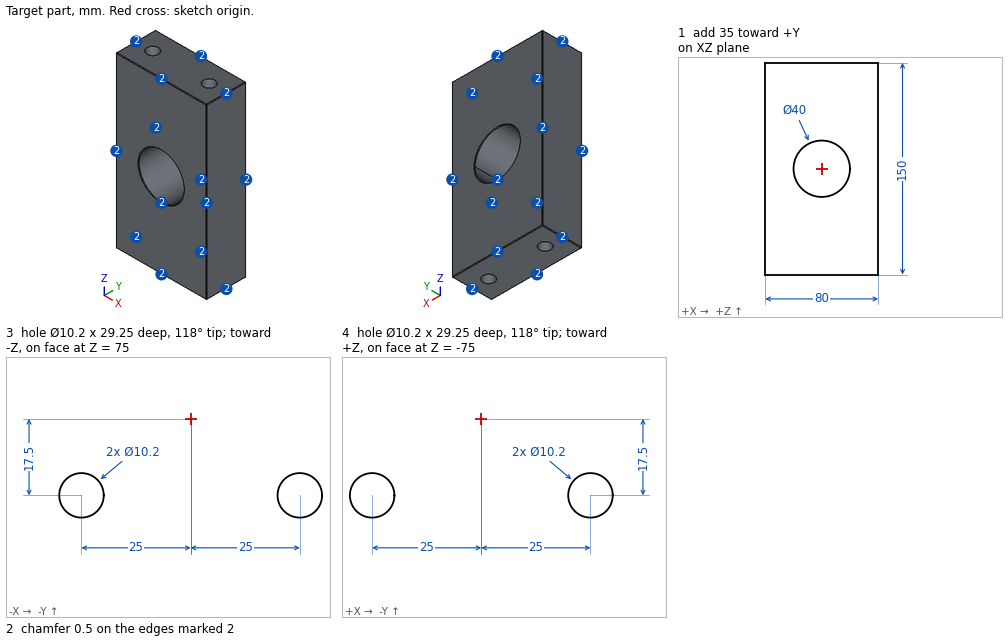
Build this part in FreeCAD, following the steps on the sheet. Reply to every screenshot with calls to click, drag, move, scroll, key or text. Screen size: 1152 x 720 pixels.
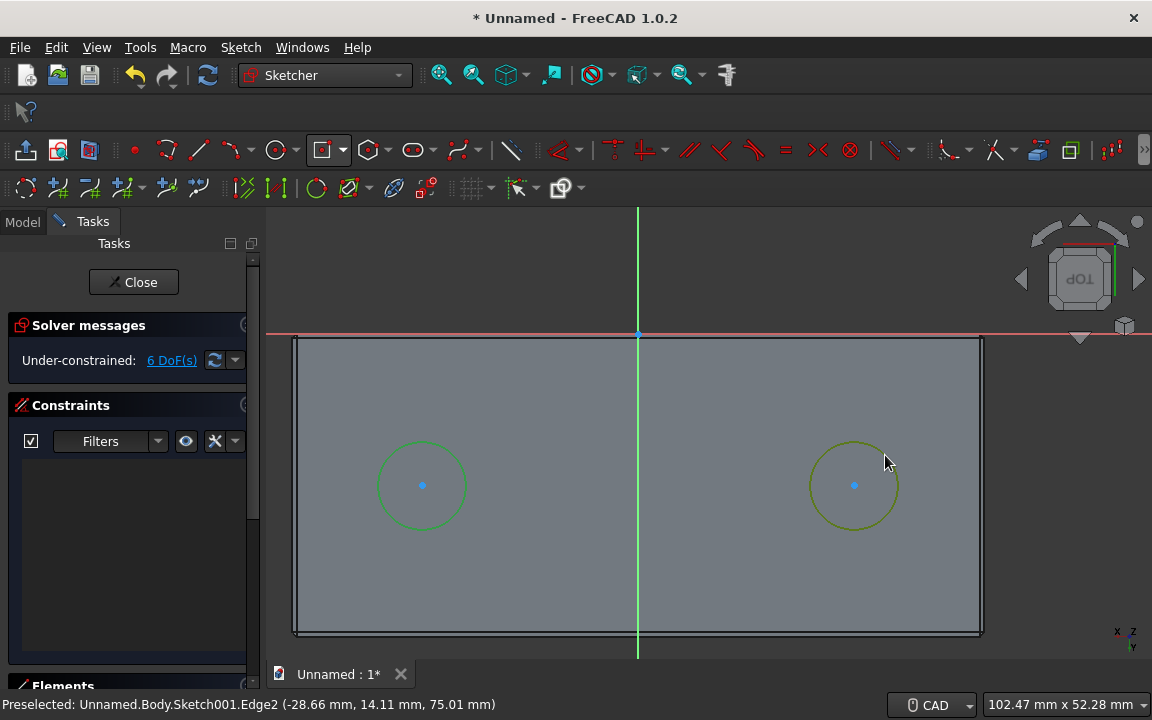
key(e)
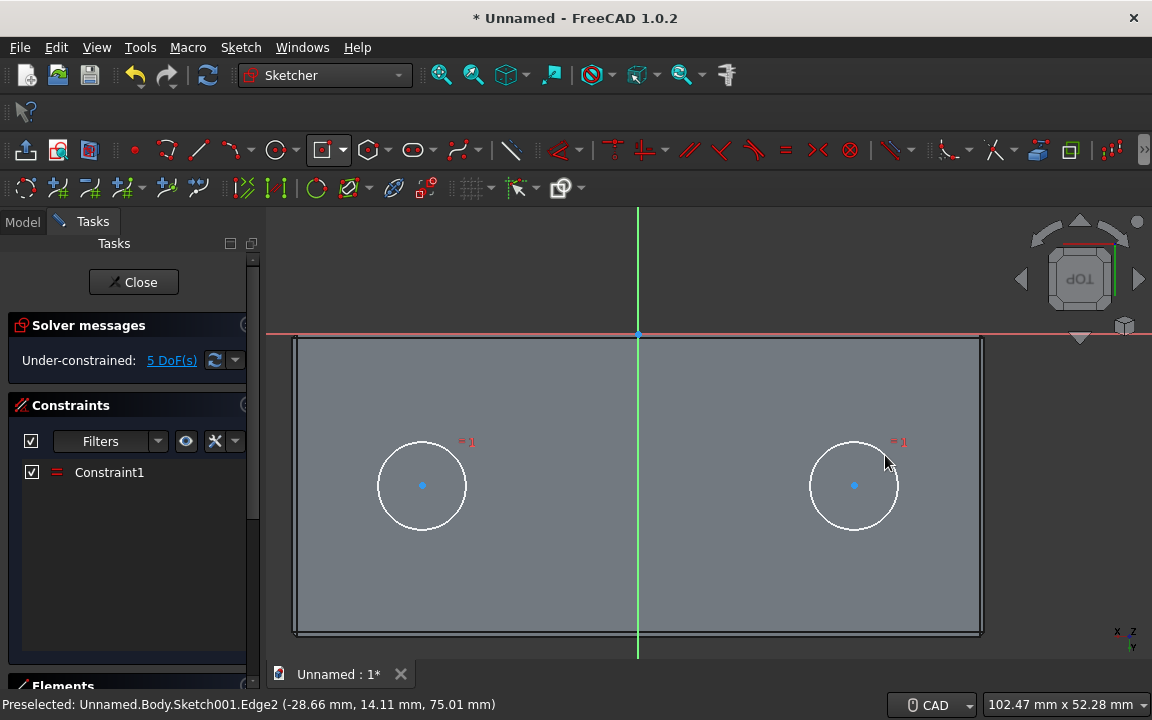
click(422, 486)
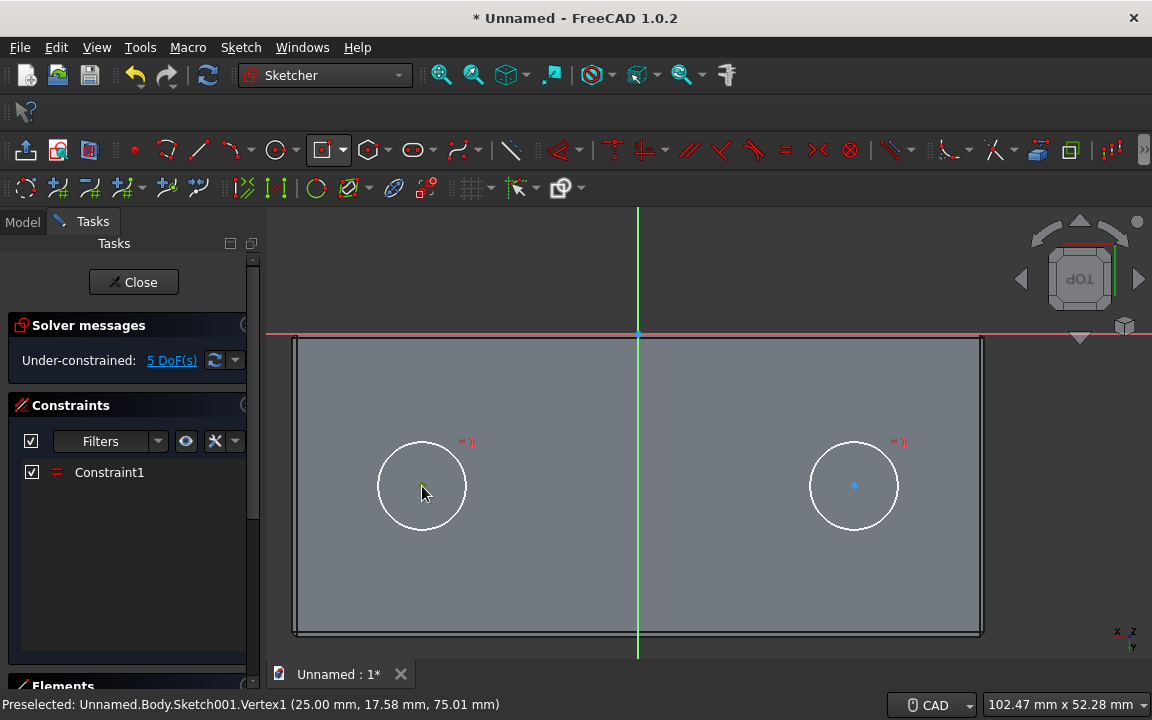
click(854, 486)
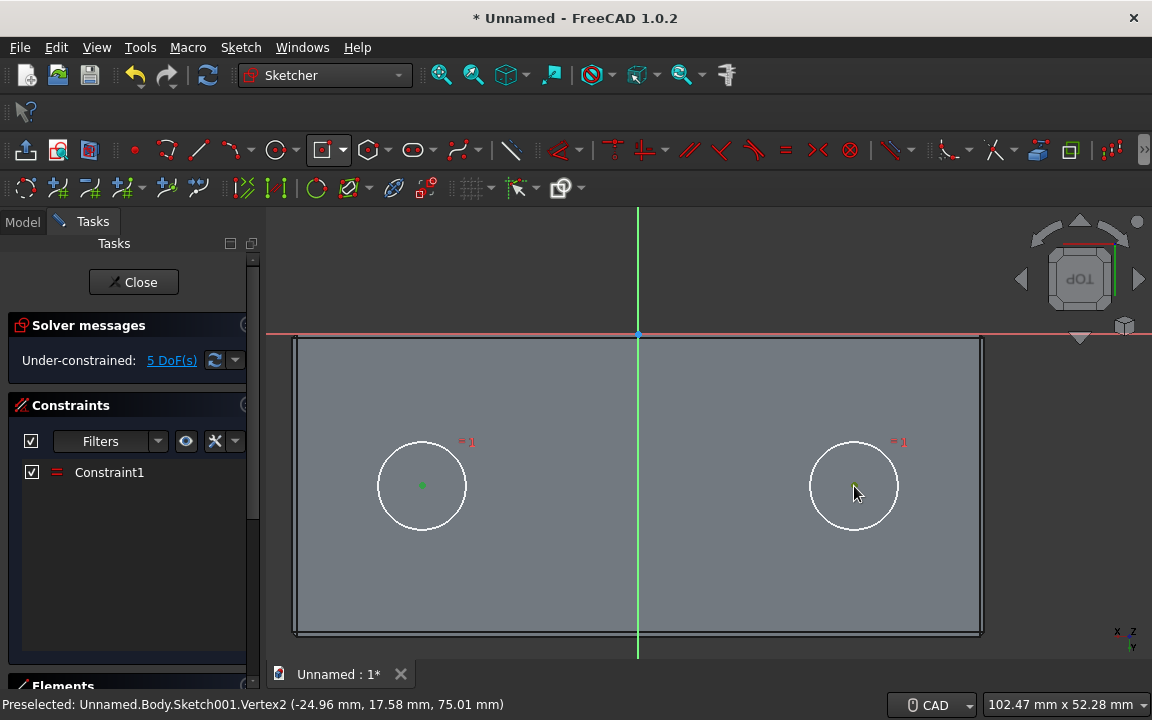
key(h)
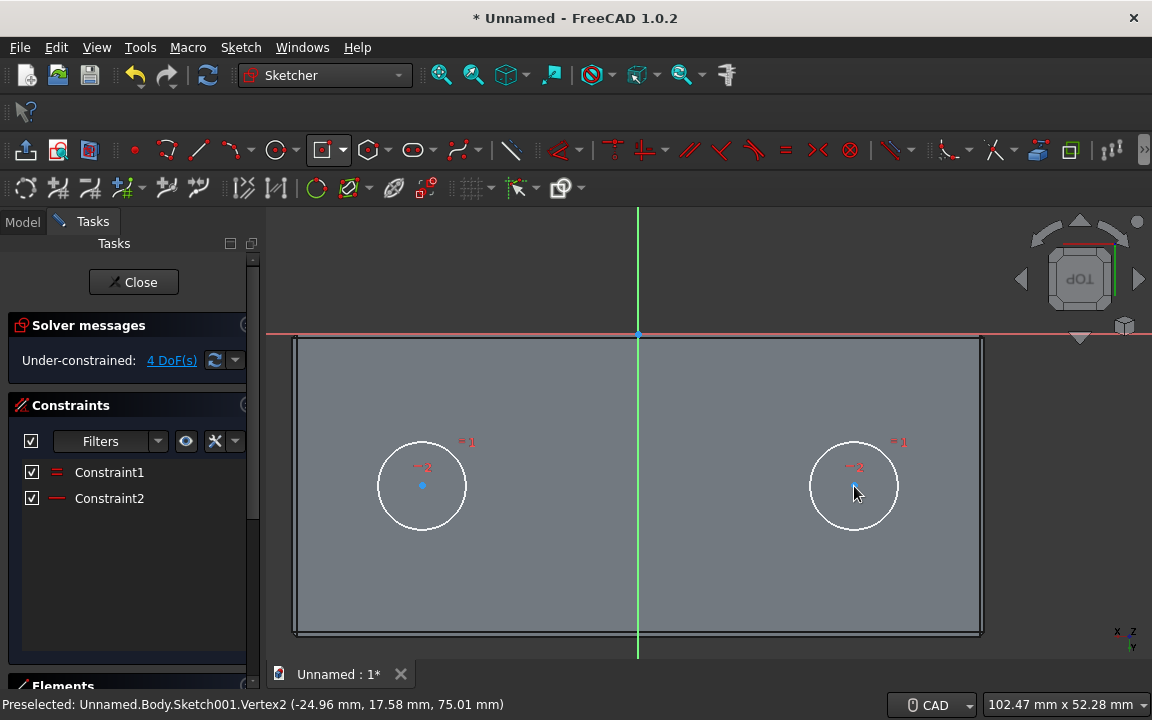
key(d)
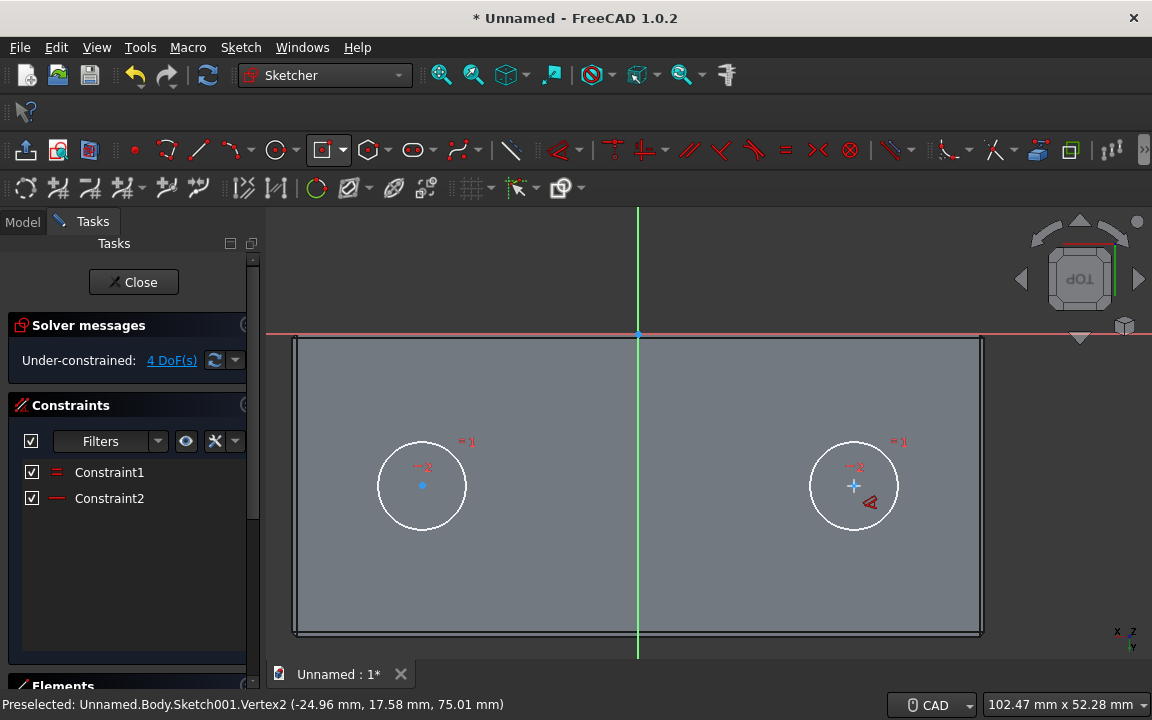
click(453, 455)
click(476, 432)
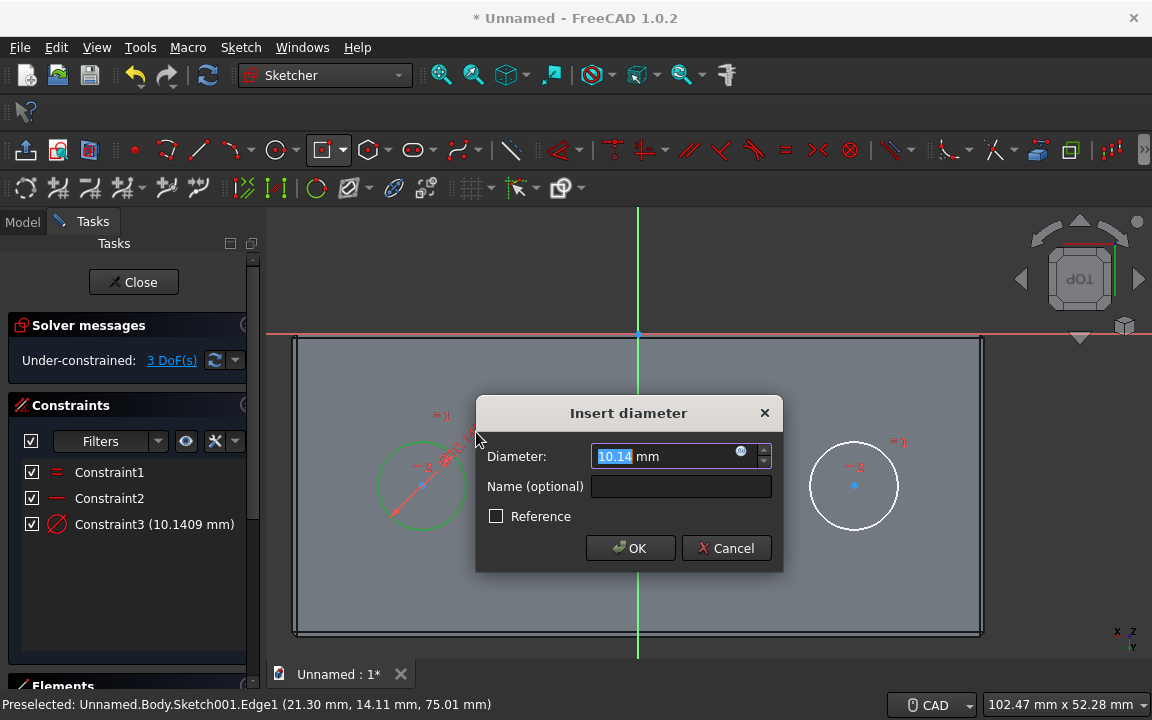
text(10.2)
key(Return)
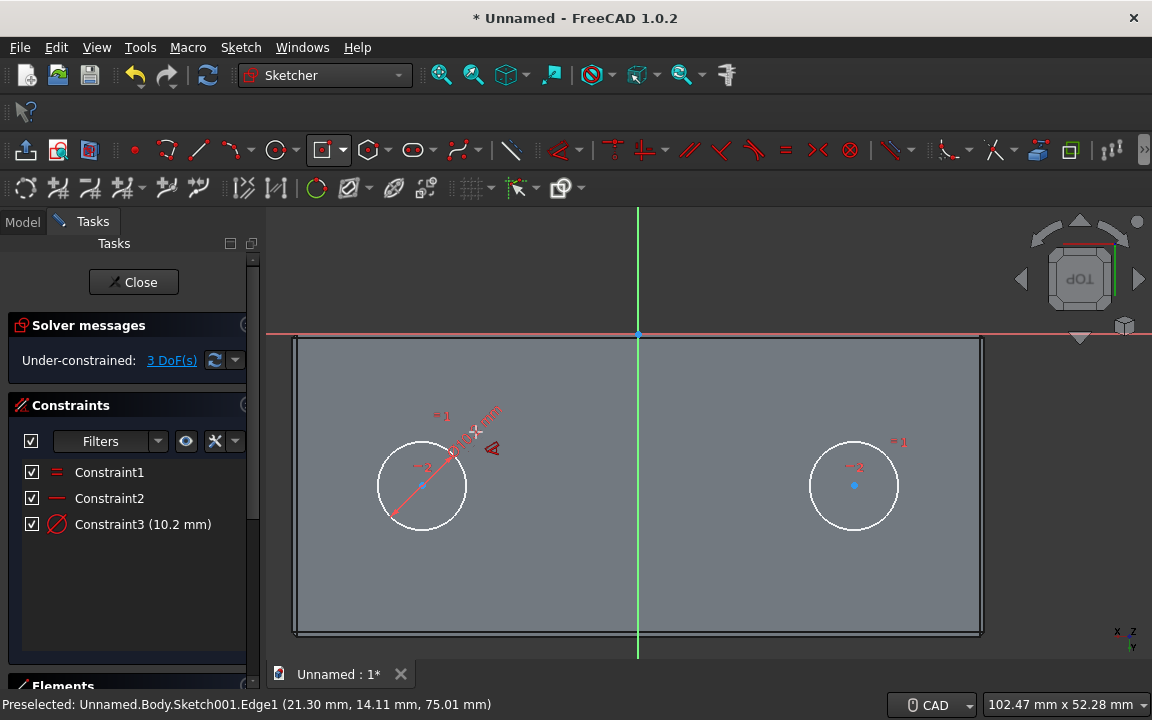
click(422, 486)
click(530, 300)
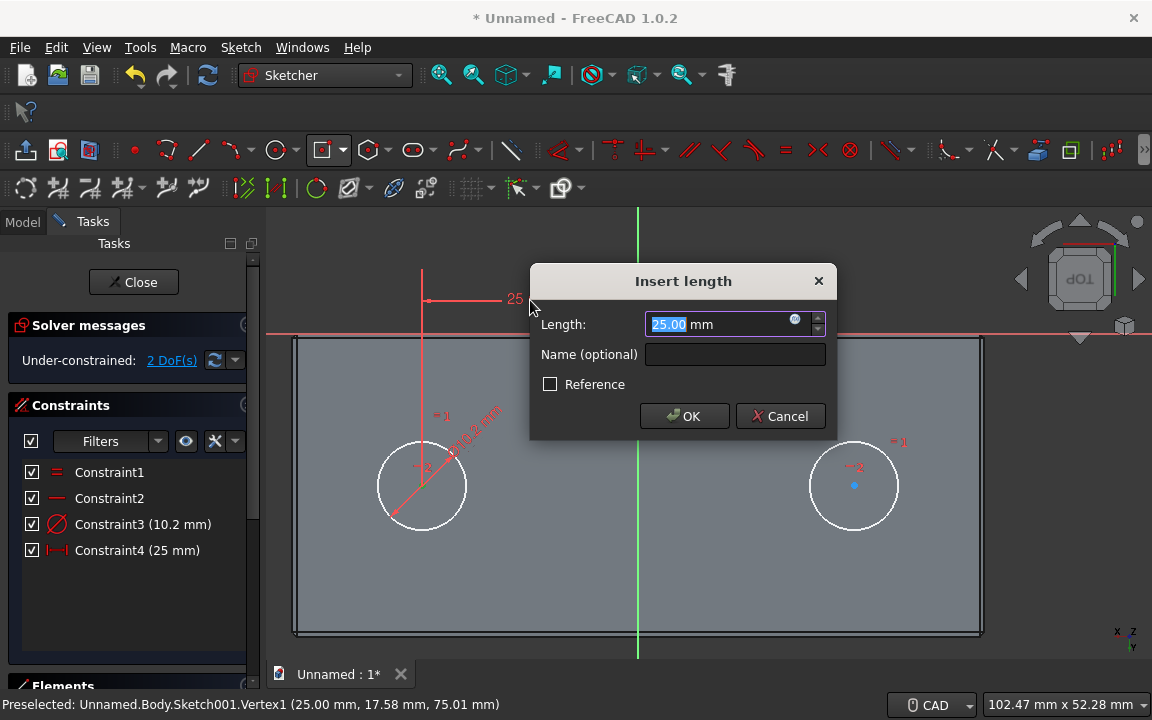
text(25)
key(Return)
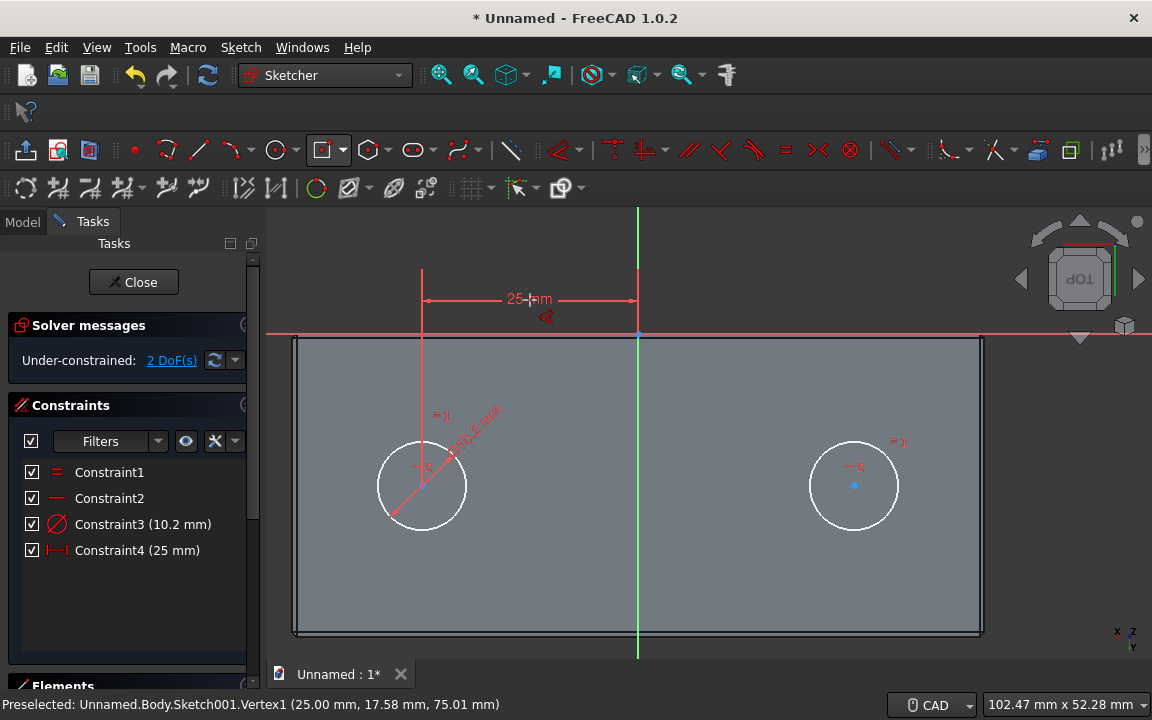
click(854, 486)
click(746, 300)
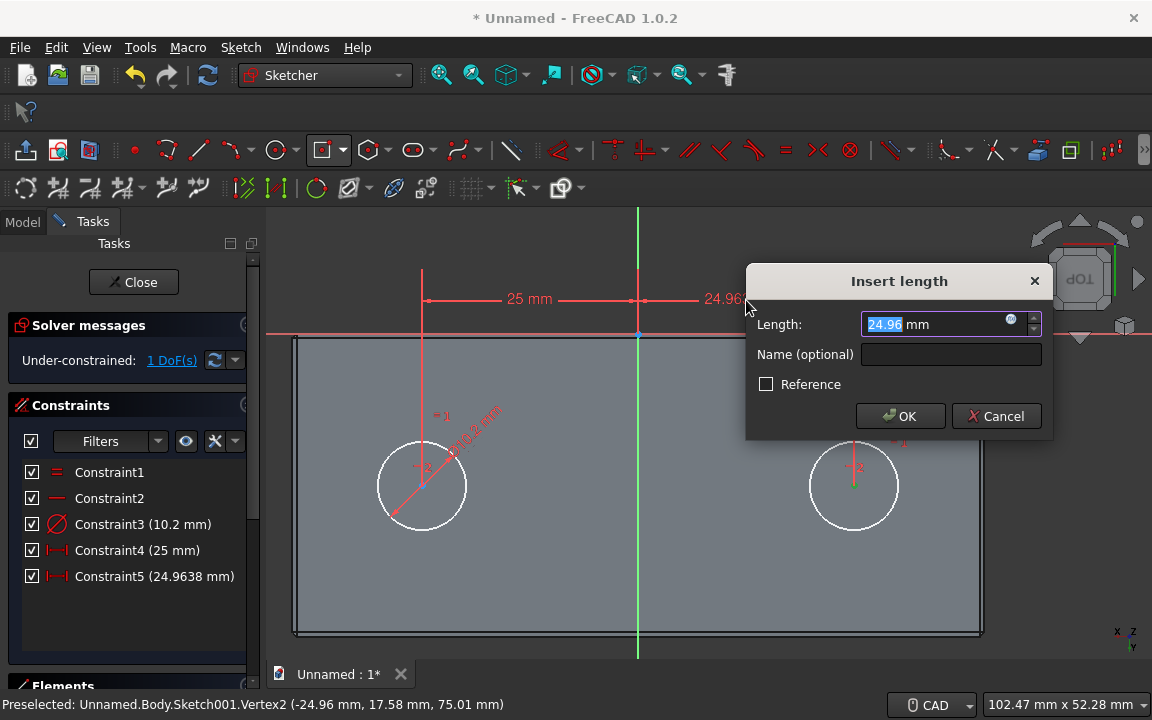
text(25)
key(Return)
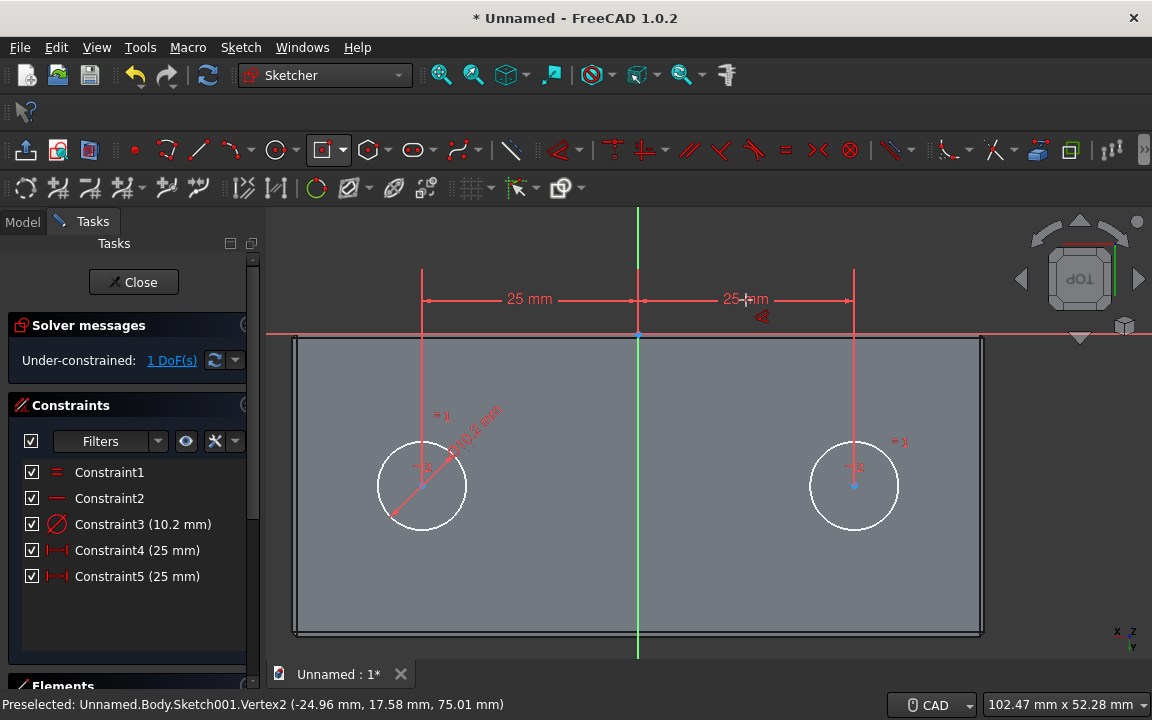
click(422, 486)
click(388, 410)